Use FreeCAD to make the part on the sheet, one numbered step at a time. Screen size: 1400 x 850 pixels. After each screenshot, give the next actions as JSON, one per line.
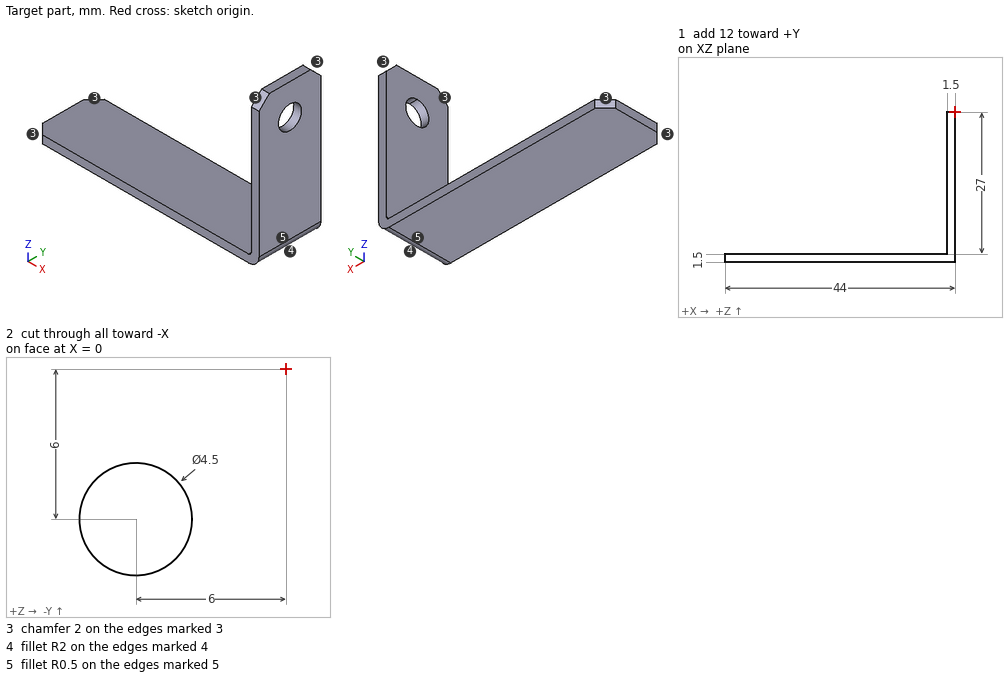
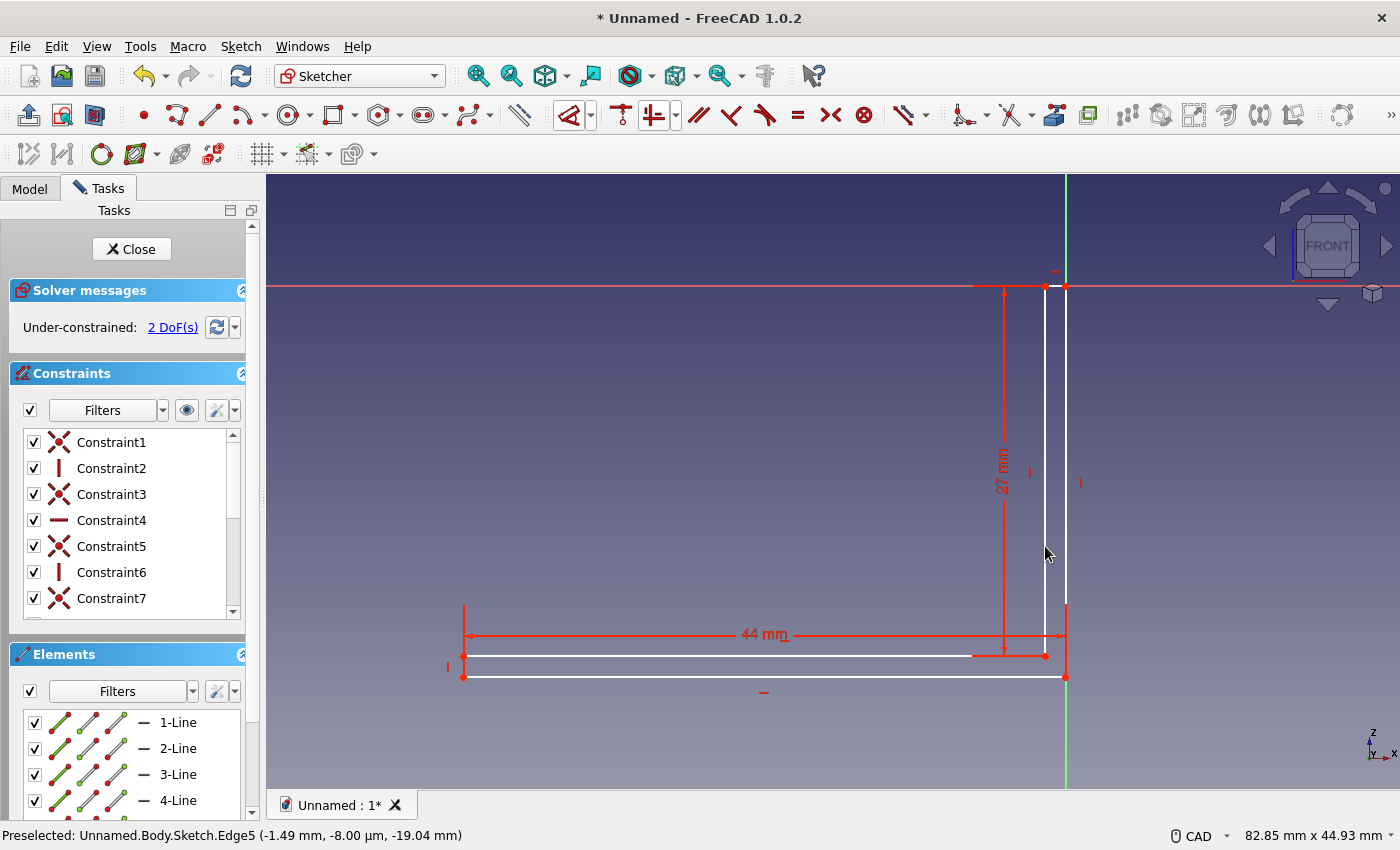
{"action": "scroll", "coordinate": [464, 667], "scroll_direction": "up", "scroll_amount": 4}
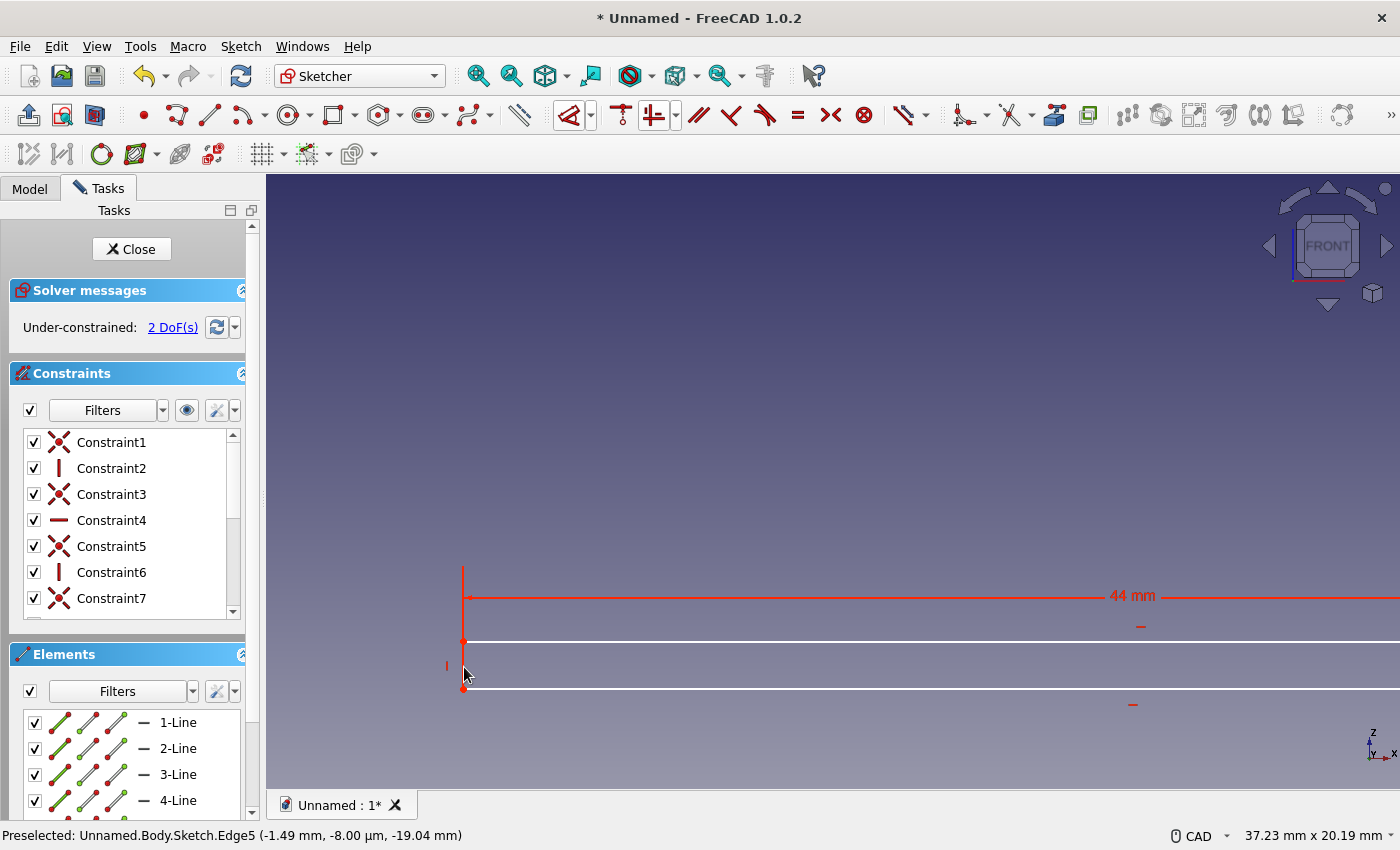
{"action": "left_click", "coordinate": [463, 665]}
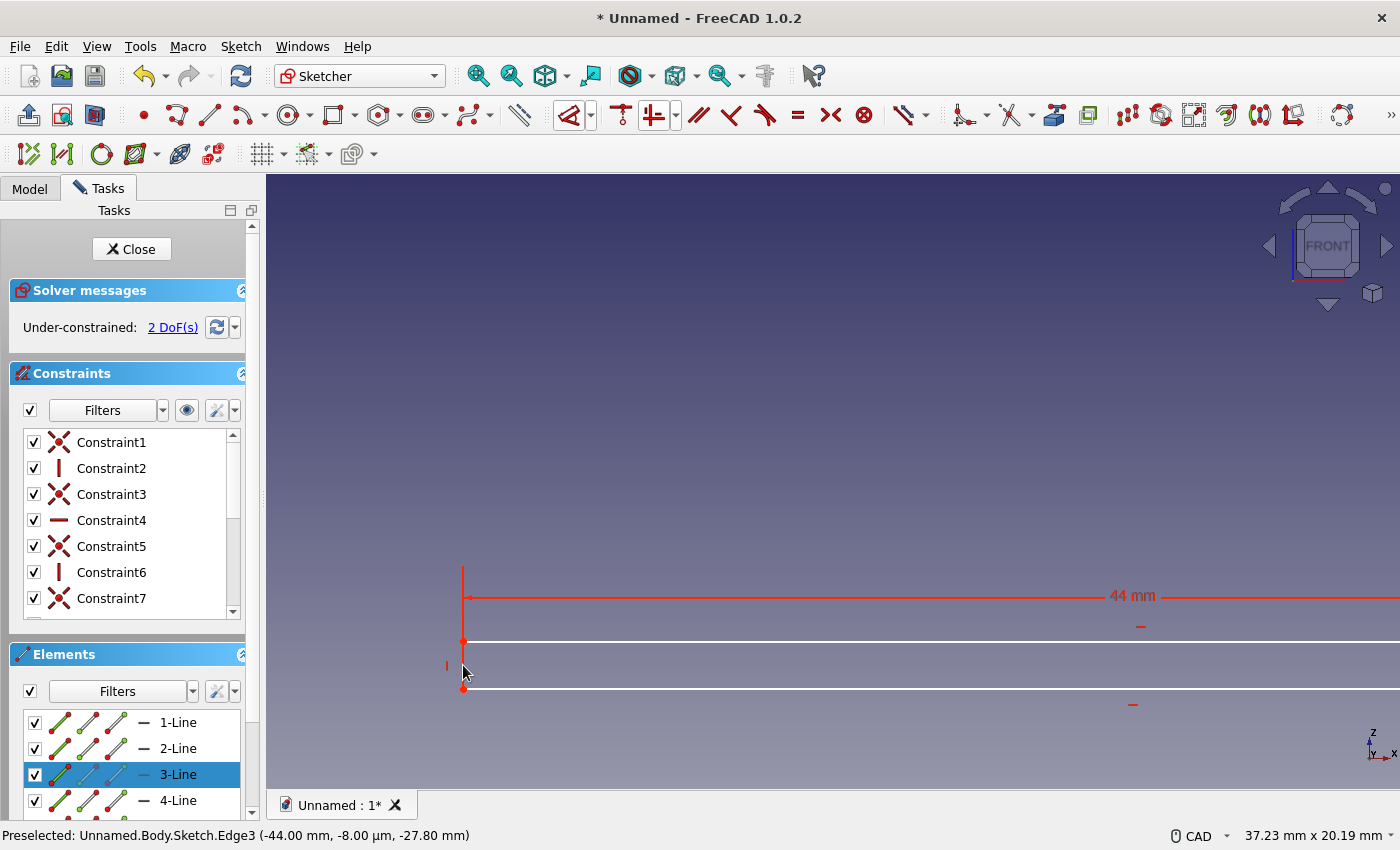
{"action": "left_click", "coordinate": [590, 116]}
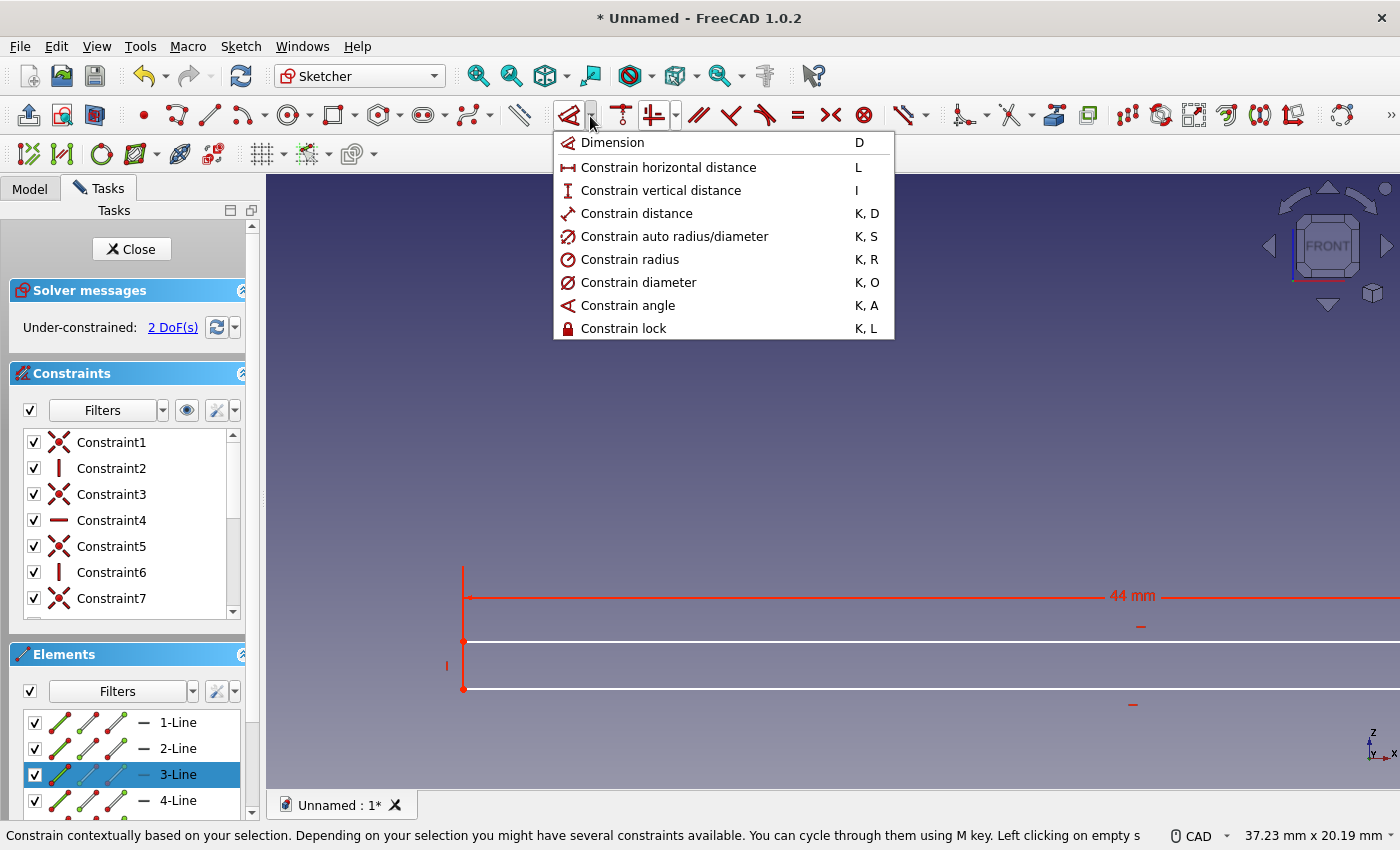
{"action": "left_click", "coordinate": [724, 190]}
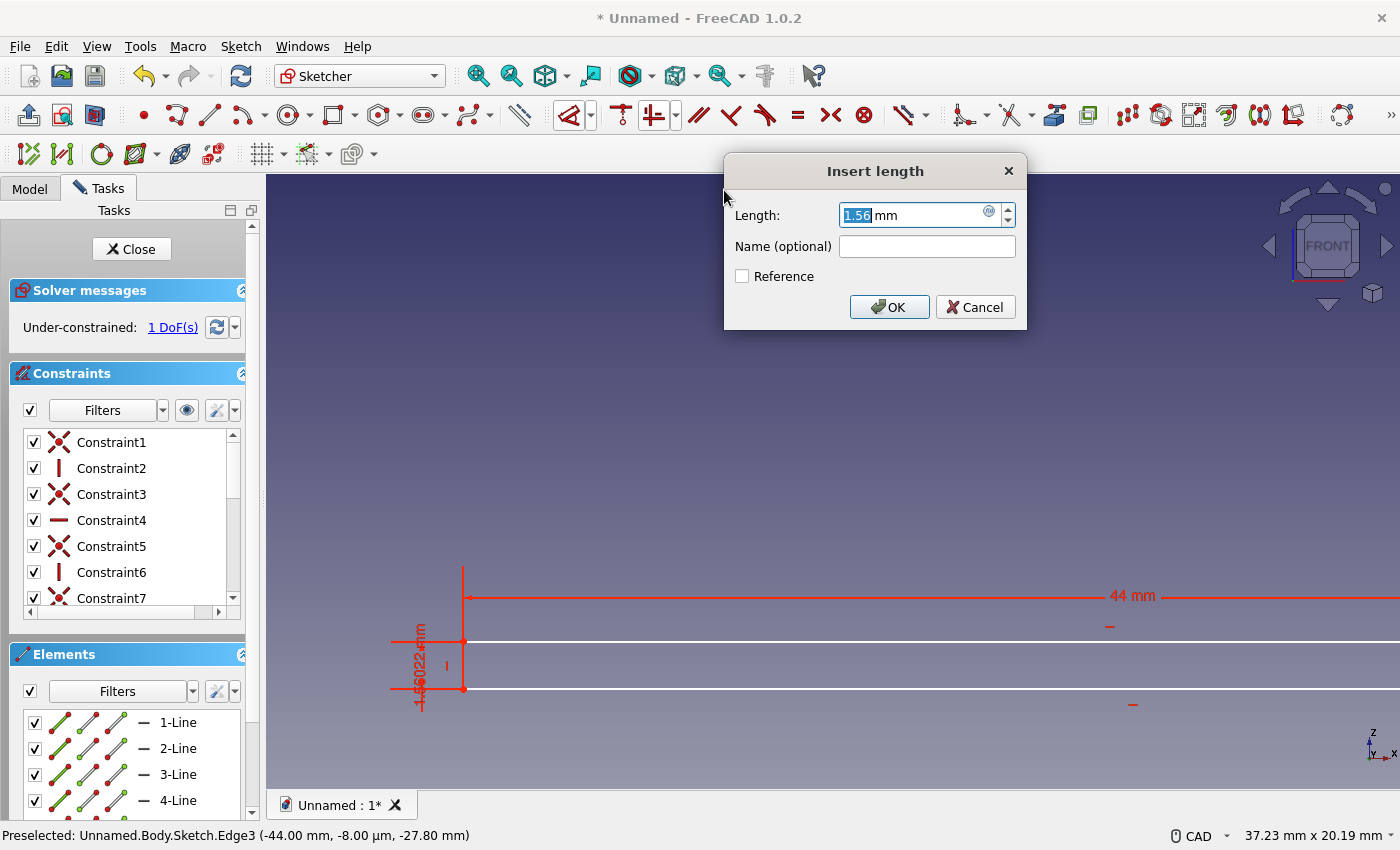
{"action": "type", "text": "1.5"}
{"action": "key", "text": "Return"}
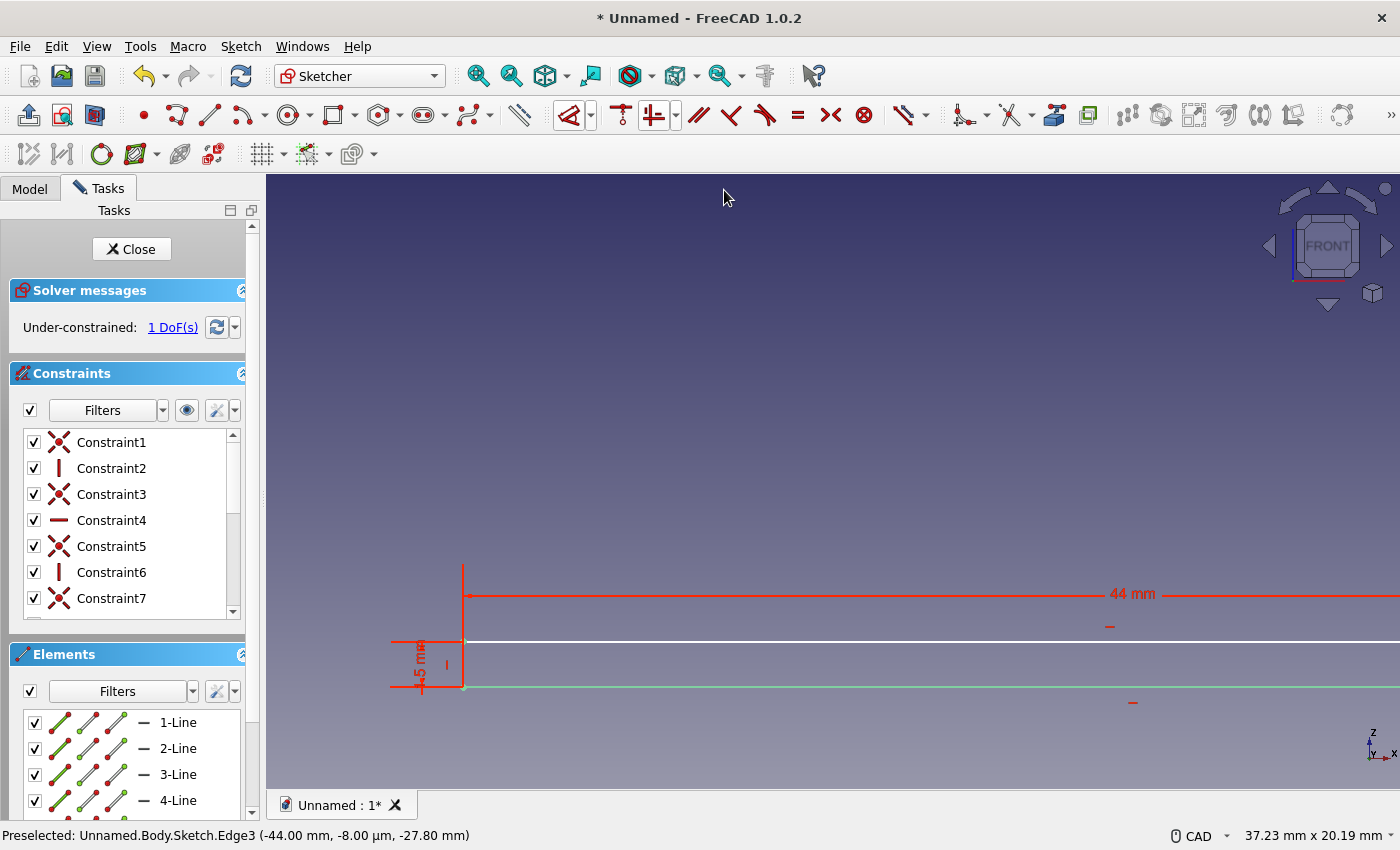
{"action": "scroll", "coordinate": [464, 668], "scroll_direction": "down", "scroll_amount": 4}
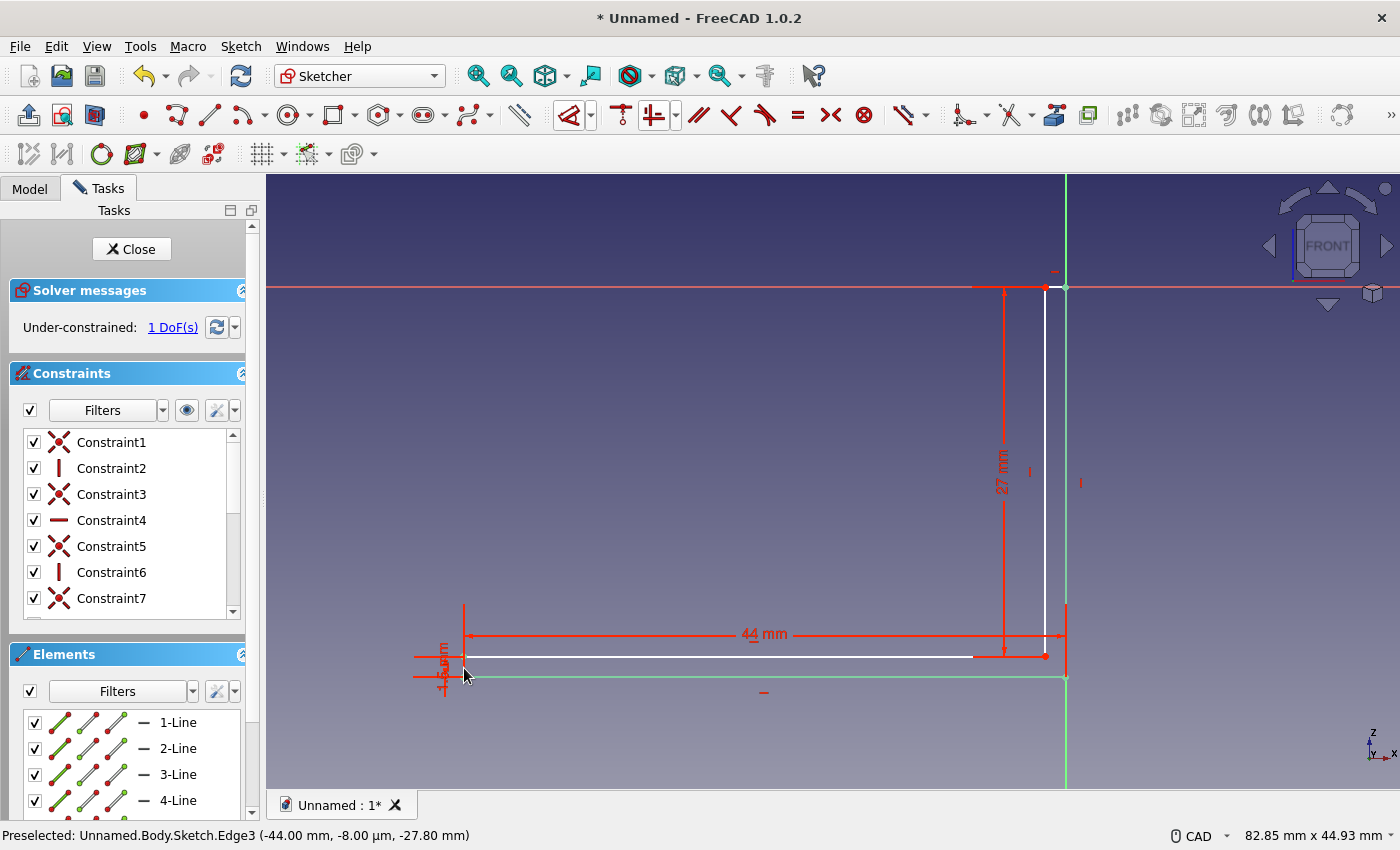
{"action": "scroll", "coordinate": [1052, 287], "scroll_direction": "up", "scroll_amount": 5}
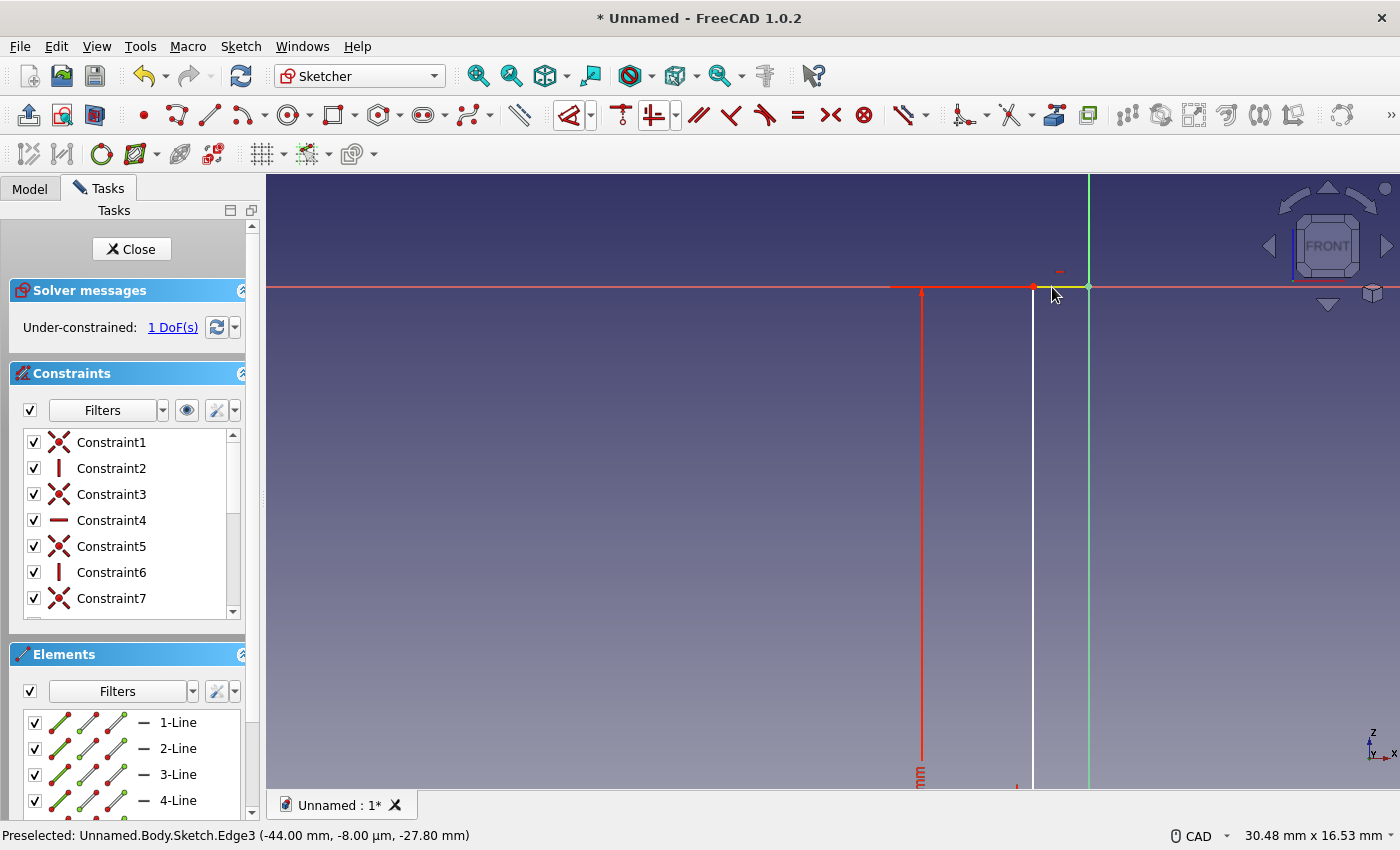
{"action": "left_click", "coordinate": [1050, 287]}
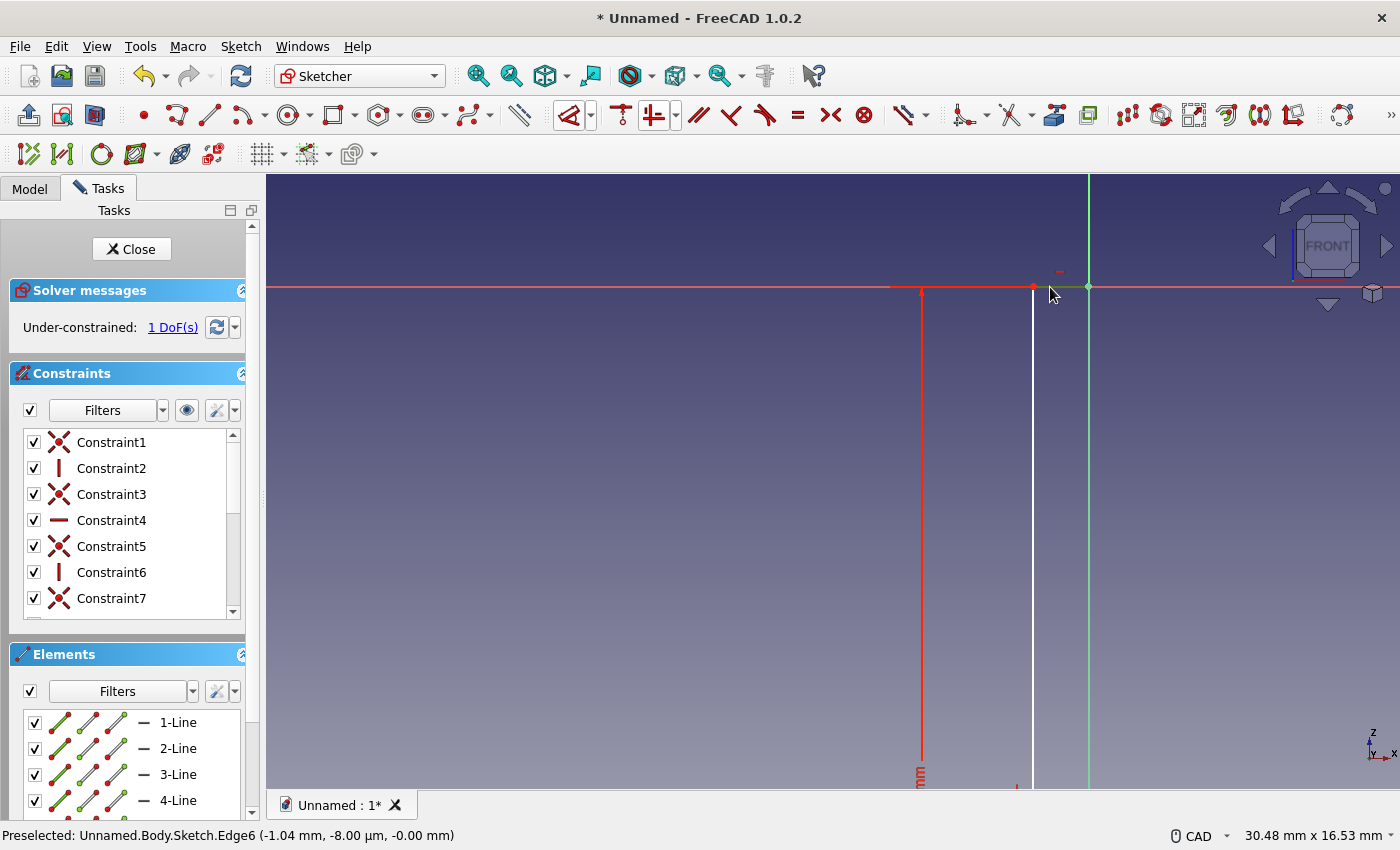
{"action": "key", "text": "l"}